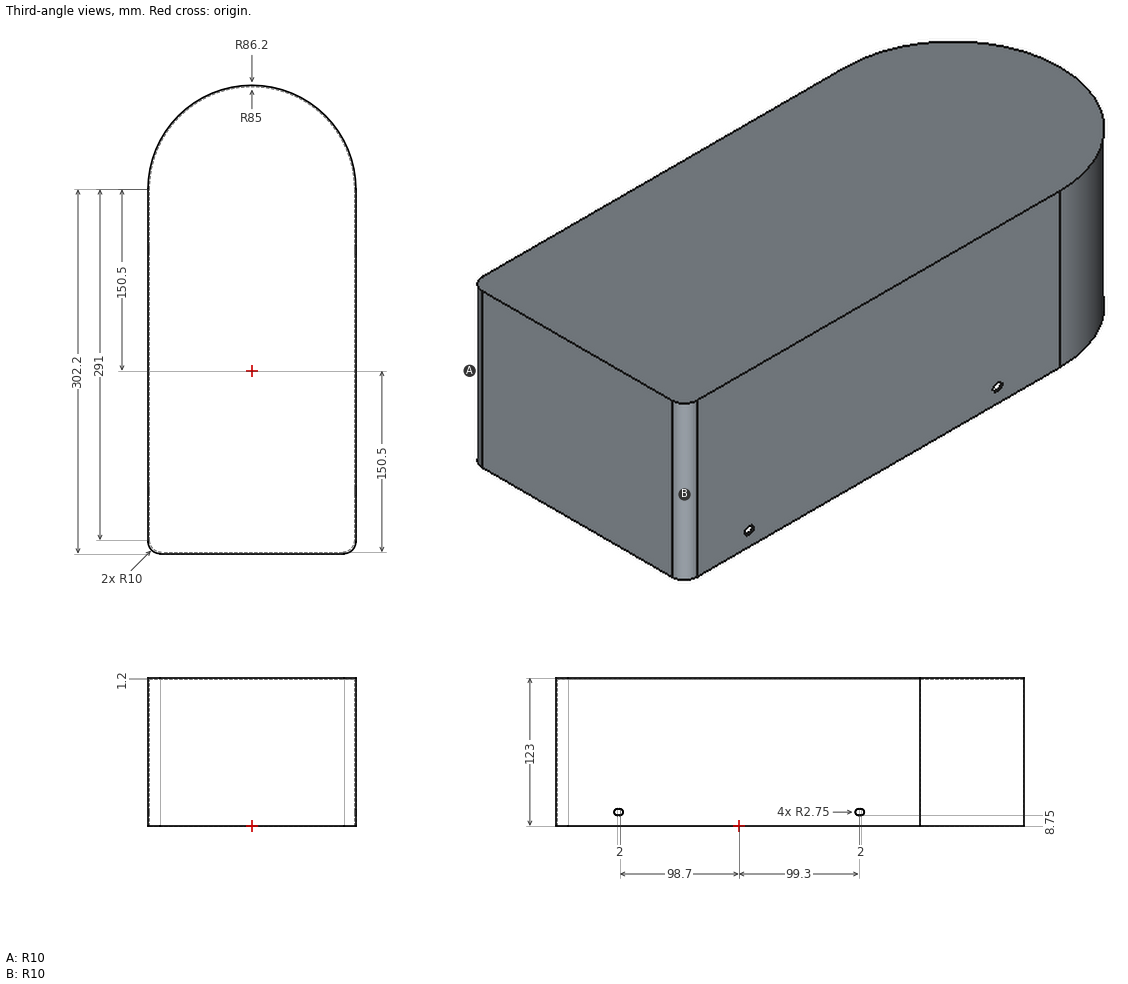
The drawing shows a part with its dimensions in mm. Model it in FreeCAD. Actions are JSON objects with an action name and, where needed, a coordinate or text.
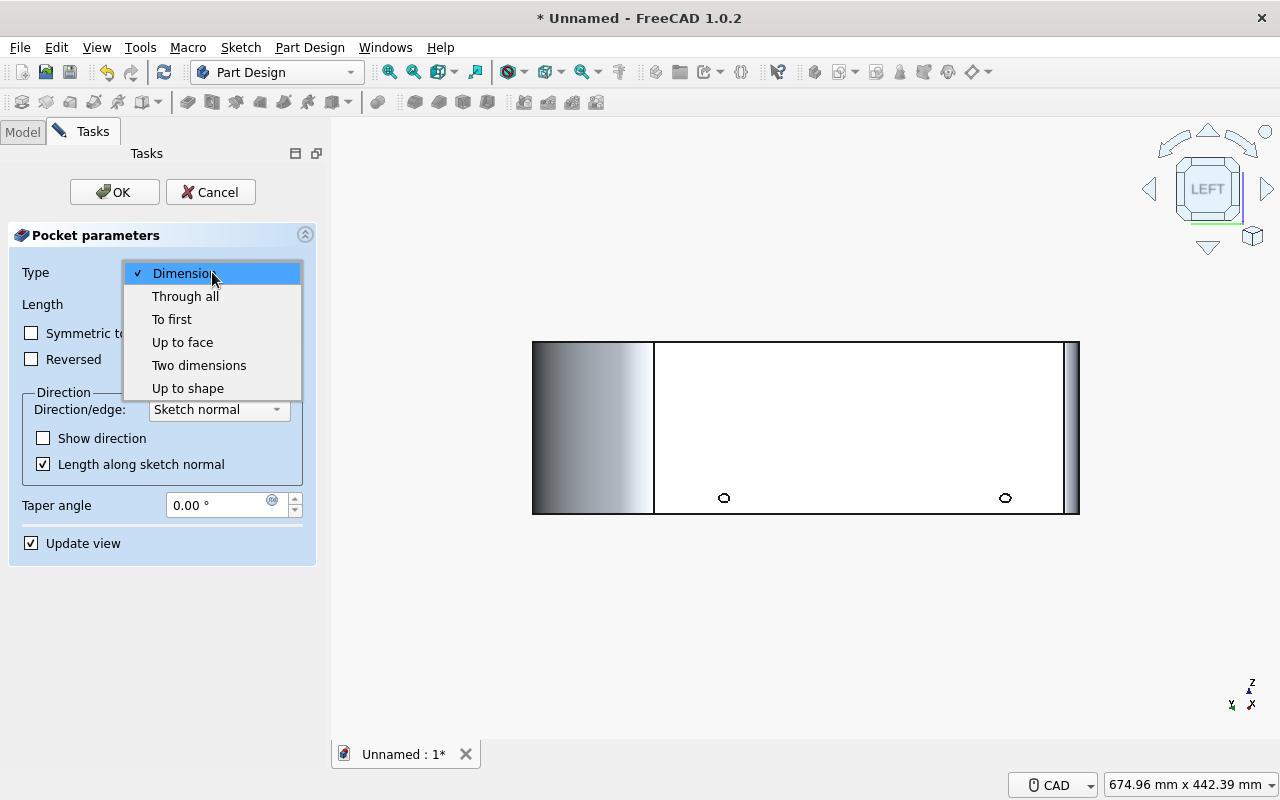
{"action": "left_click", "coordinate": [212, 296]}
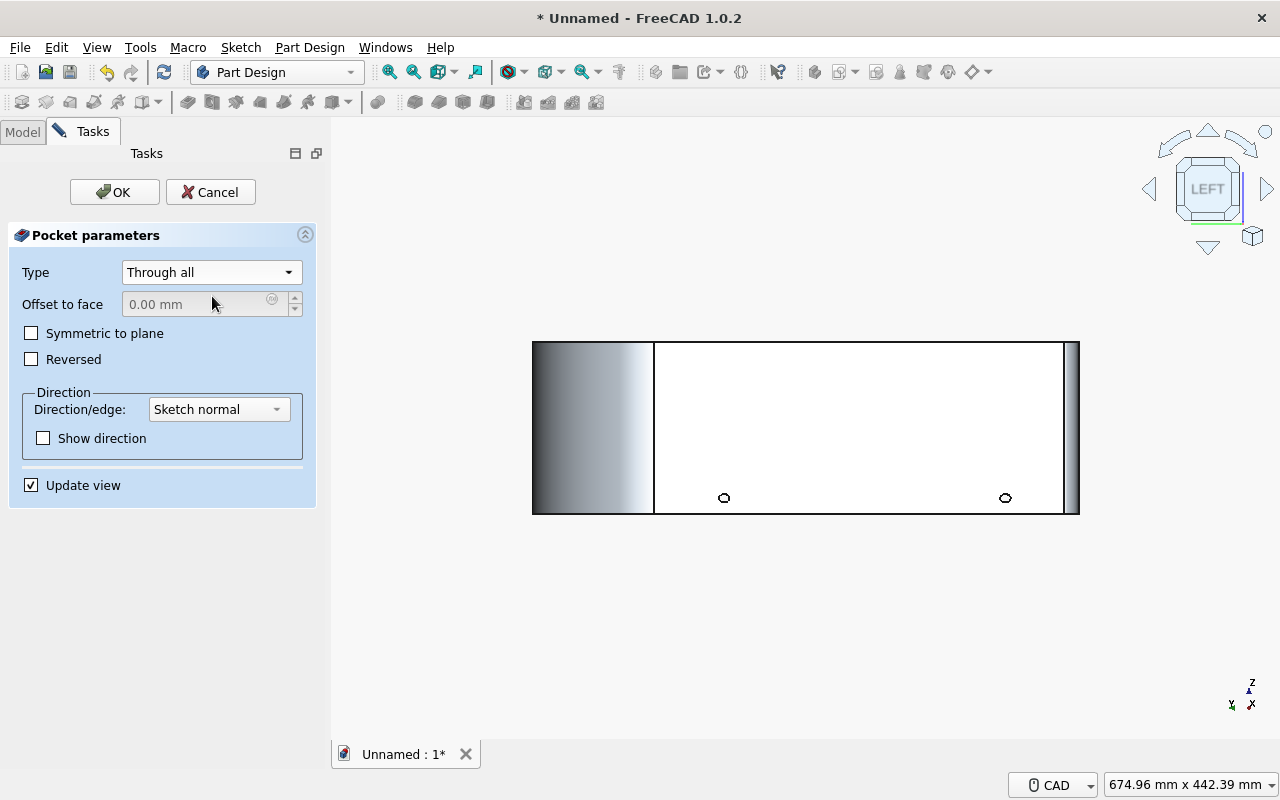
{"action": "left_click", "coordinate": [115, 192]}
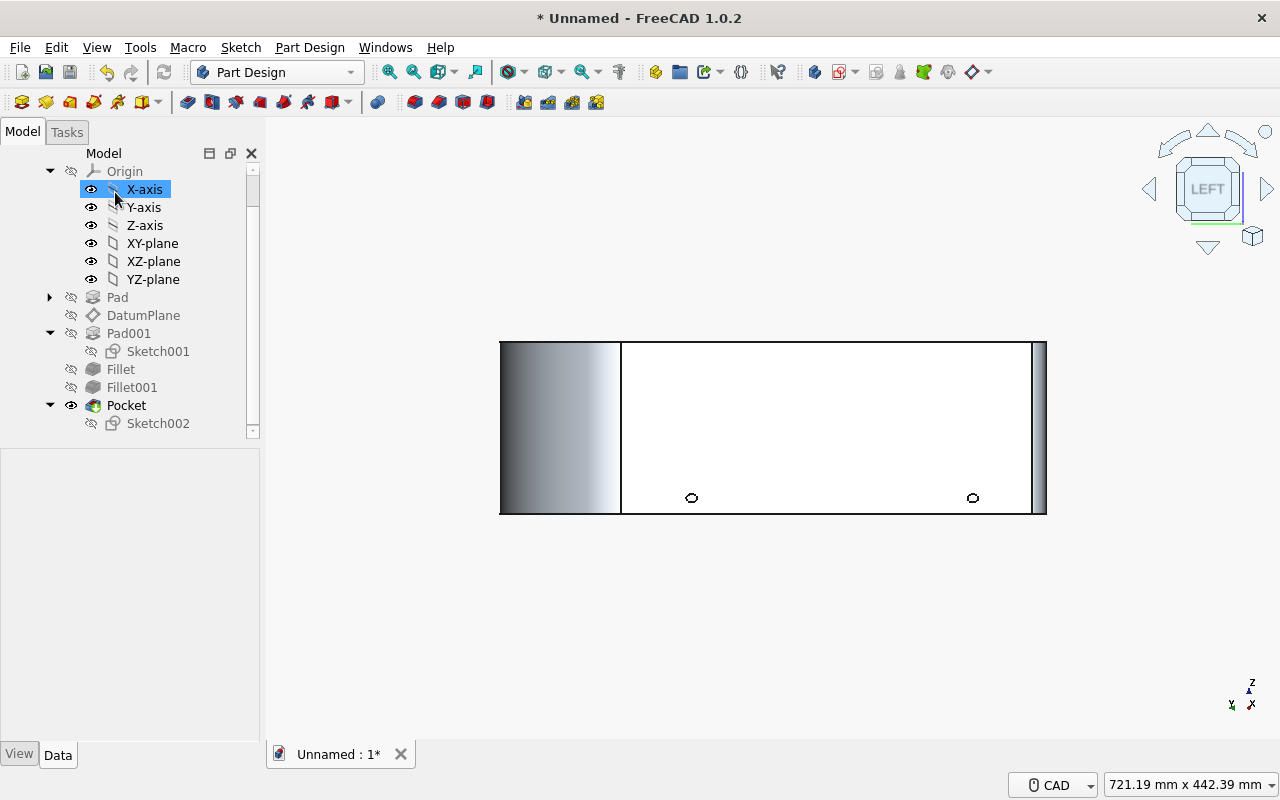
{"action": "key", "text": "0"}